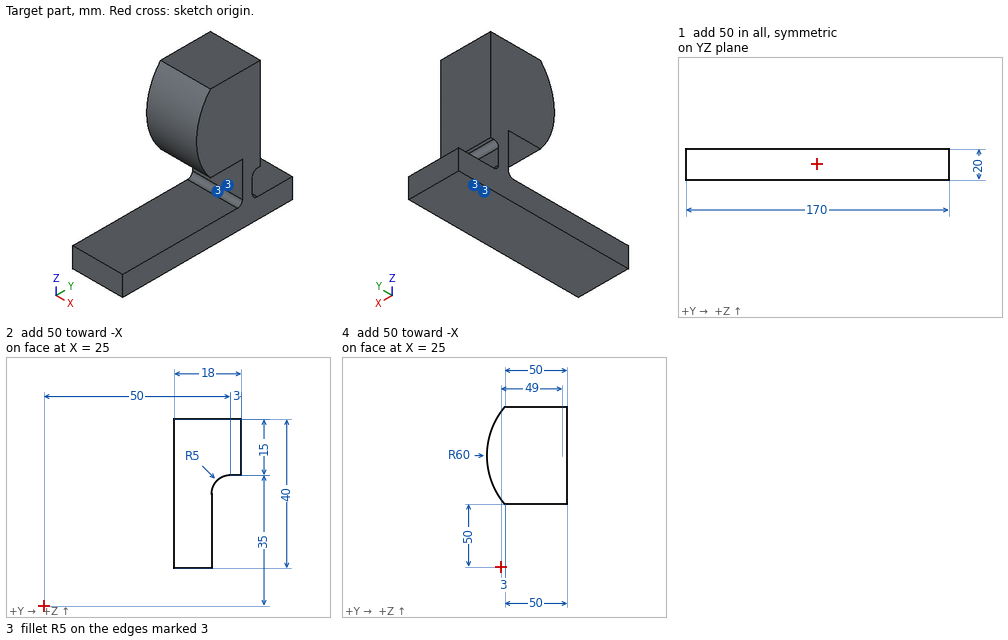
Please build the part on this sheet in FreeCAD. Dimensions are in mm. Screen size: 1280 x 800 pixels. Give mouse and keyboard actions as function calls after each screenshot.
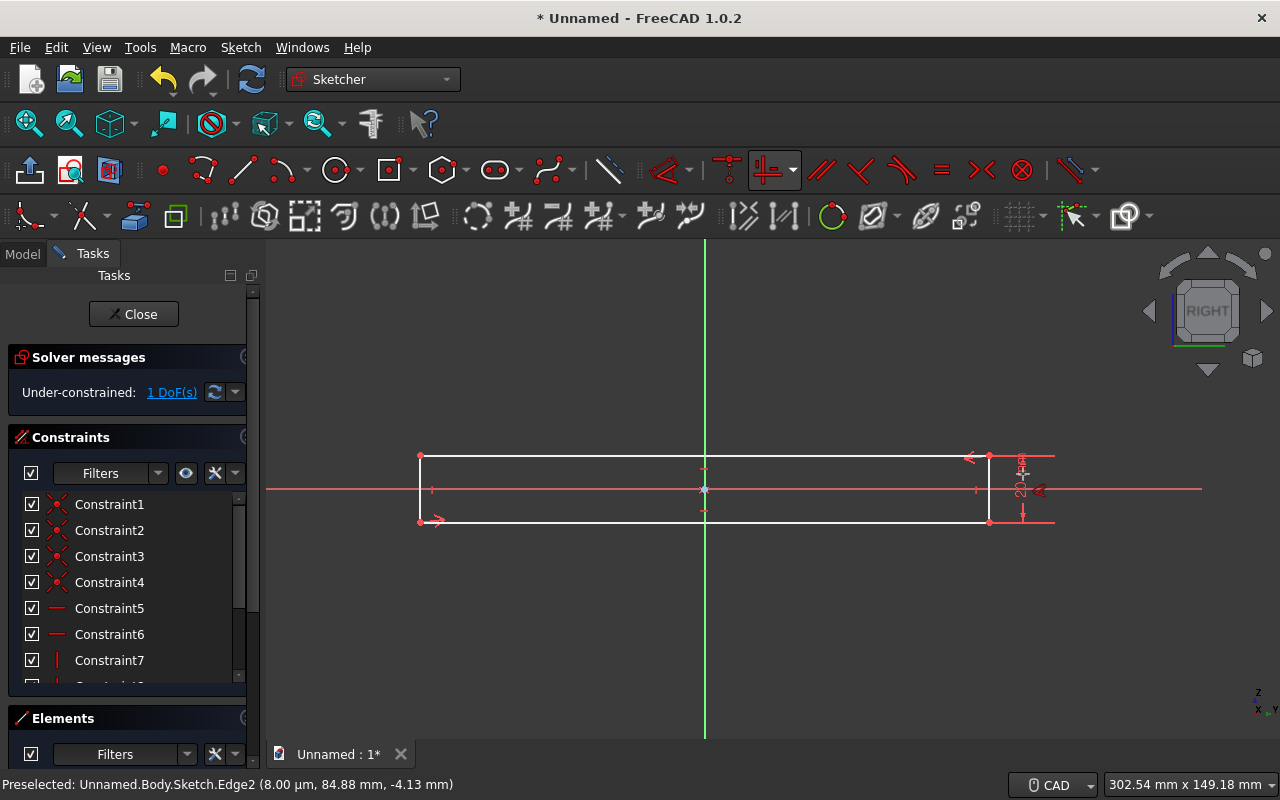
click(591, 523)
click(574, 557)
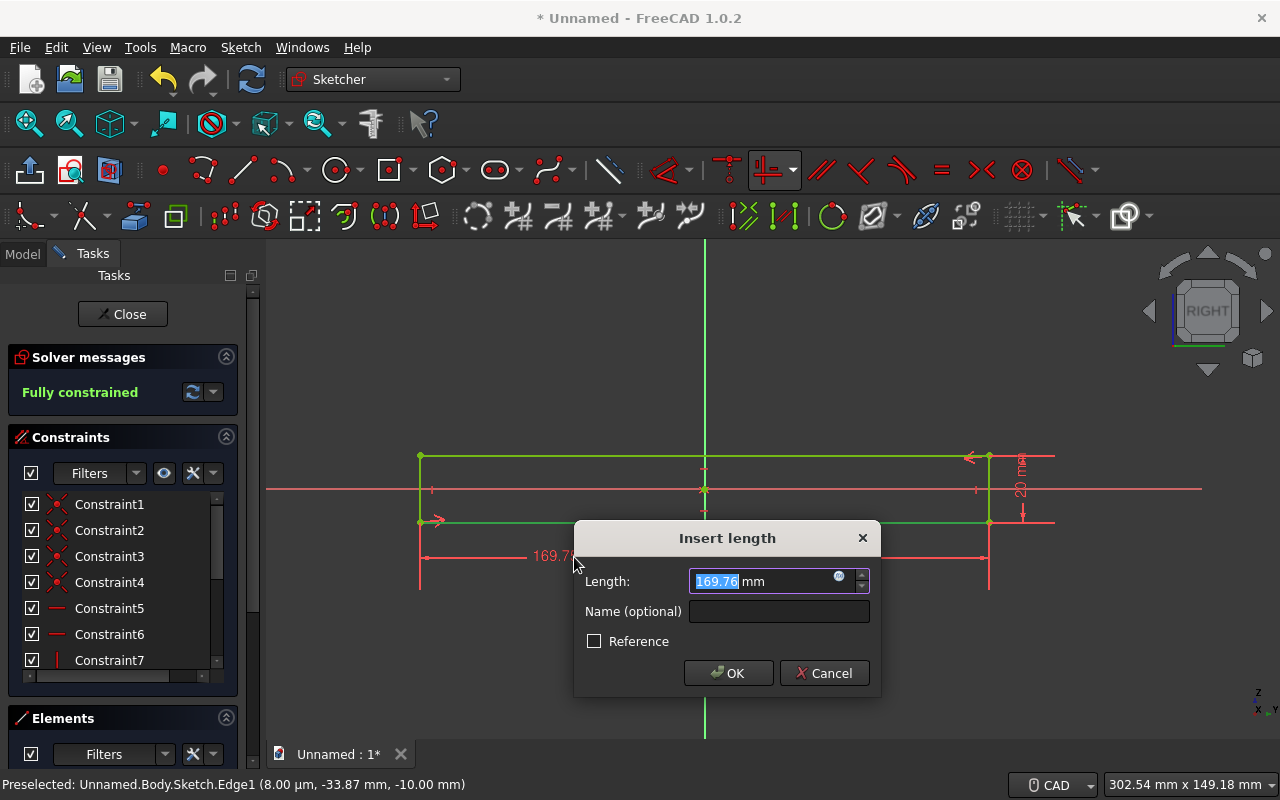
text(170)
key(Return)
key(Escape)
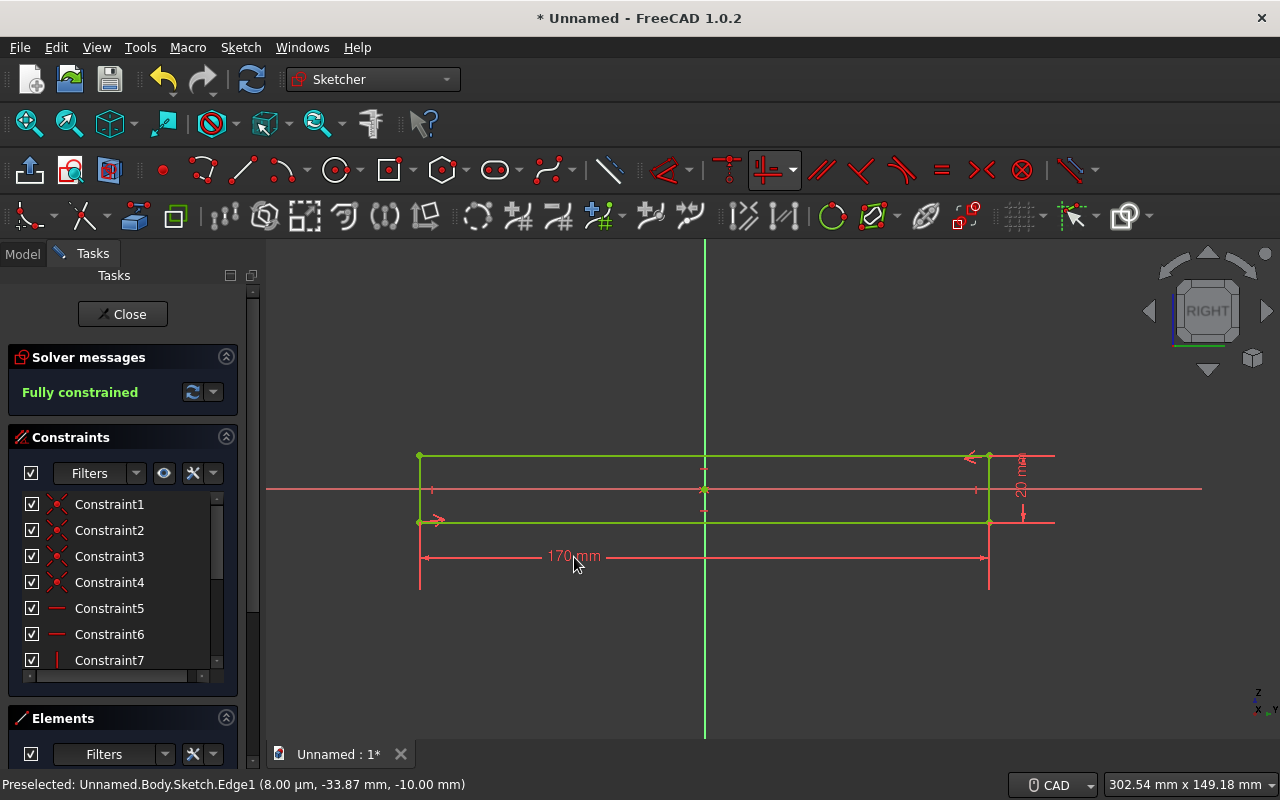
click(123, 314)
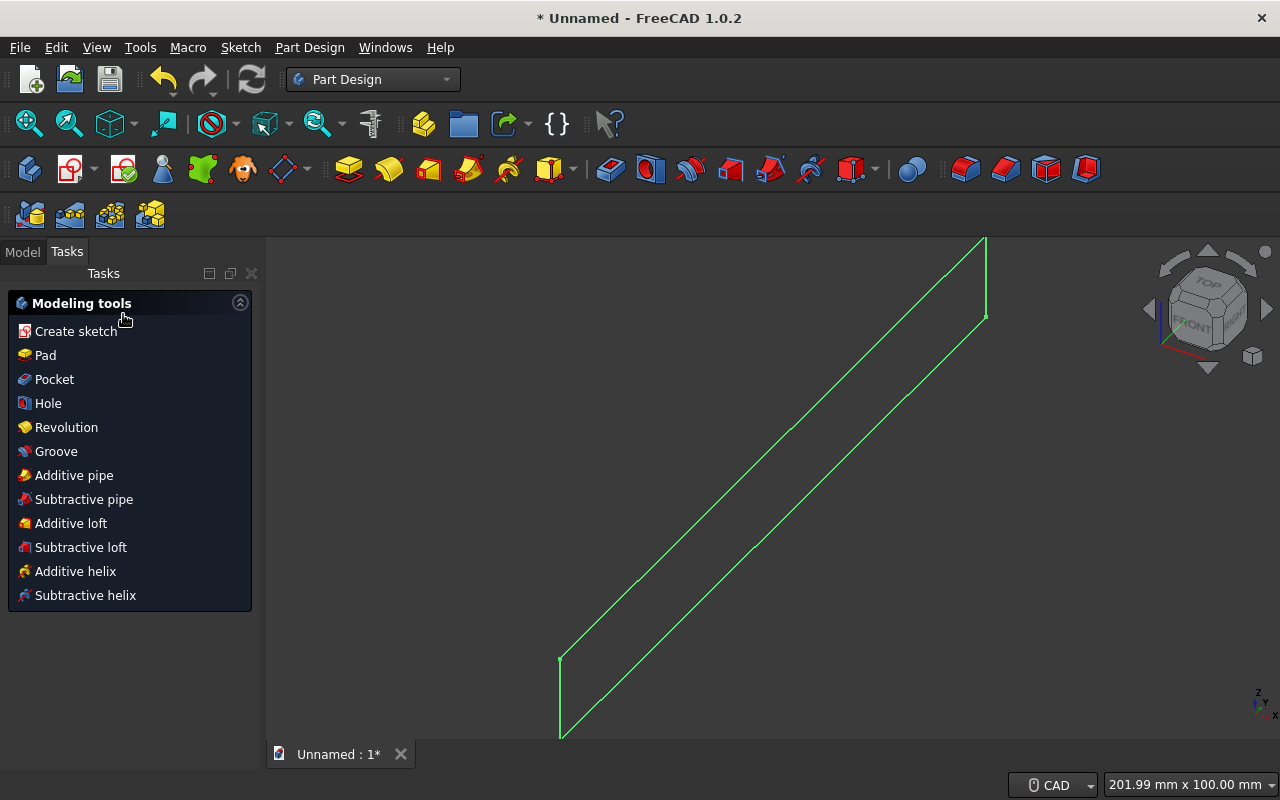
click(350, 170)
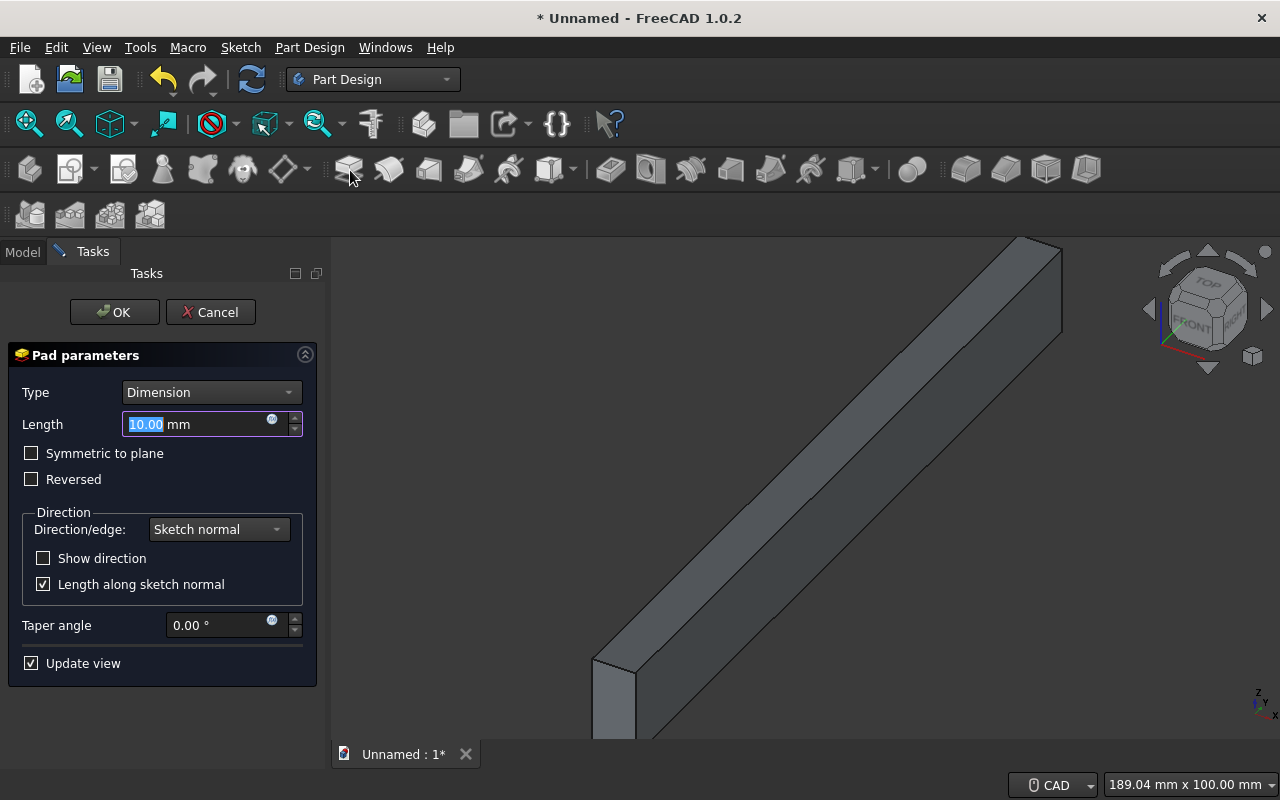
text(50)
key(Tab)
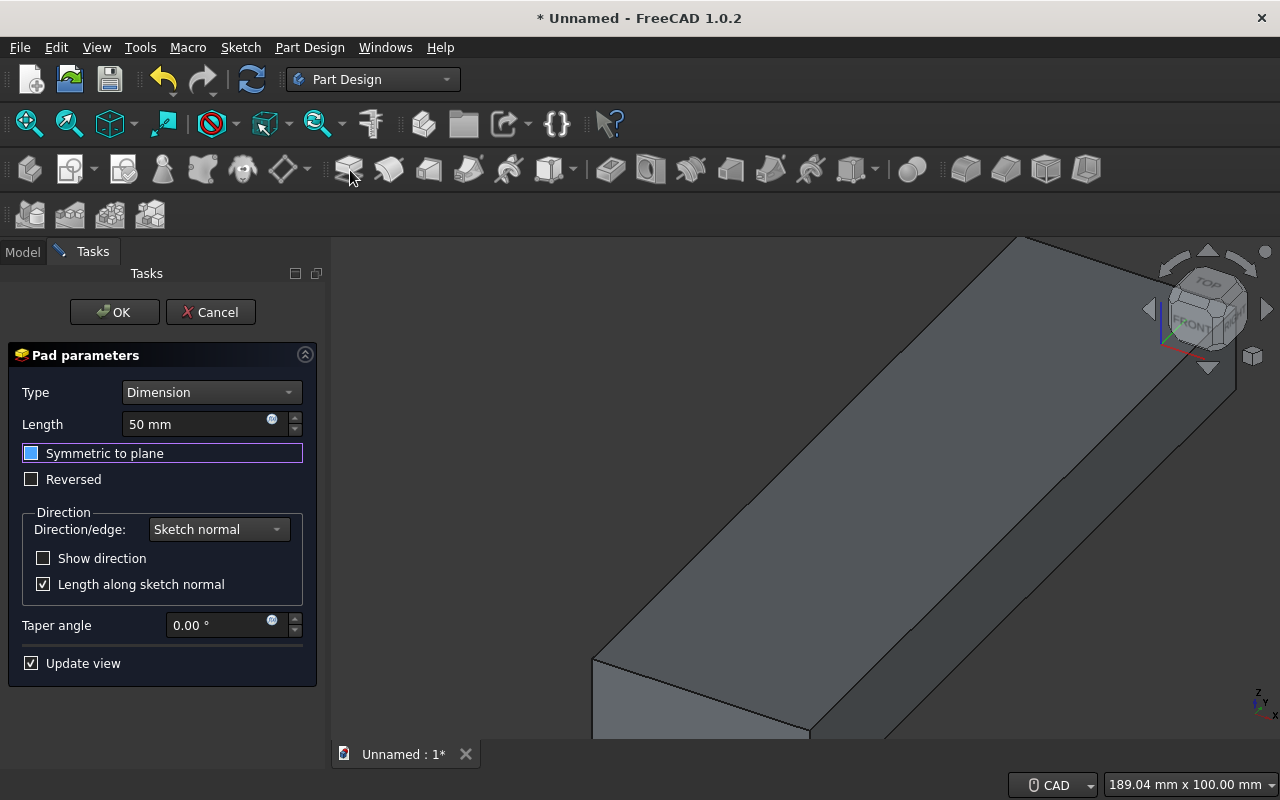
click(30, 453)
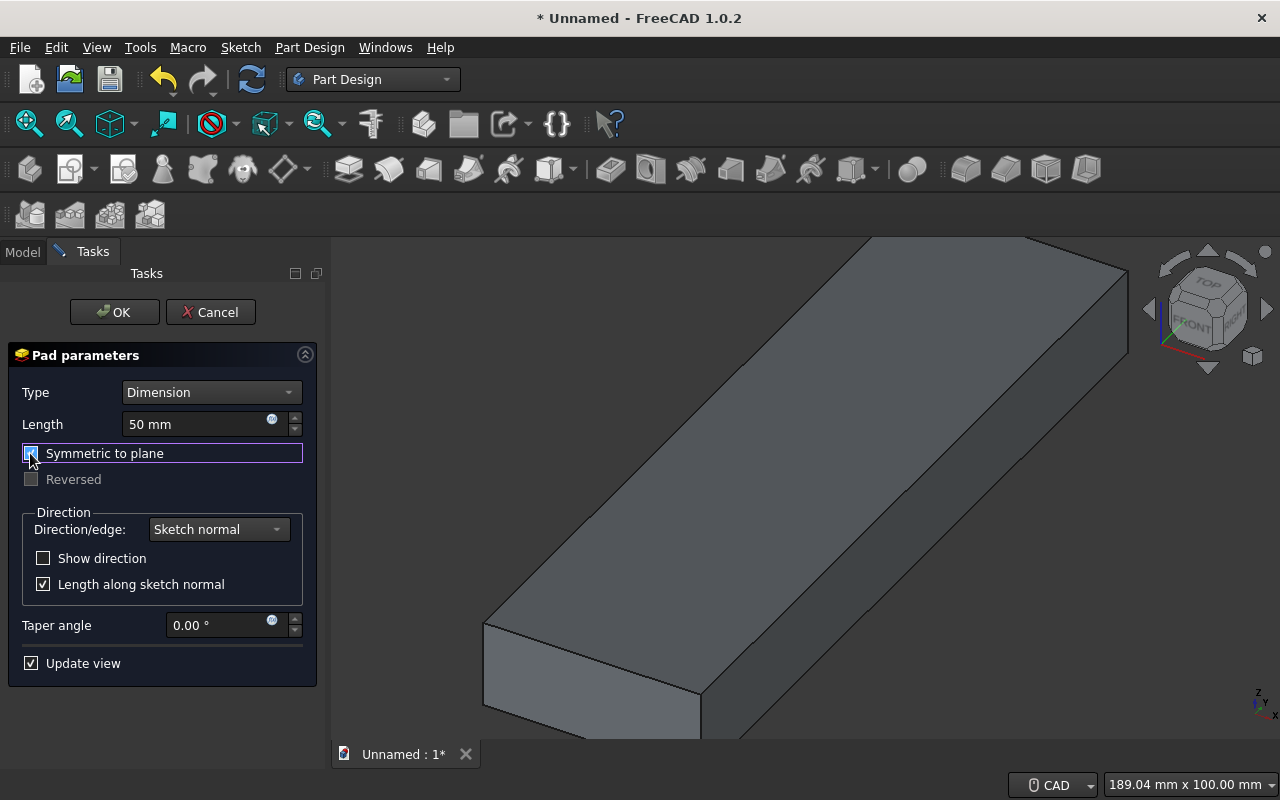
click(115, 312)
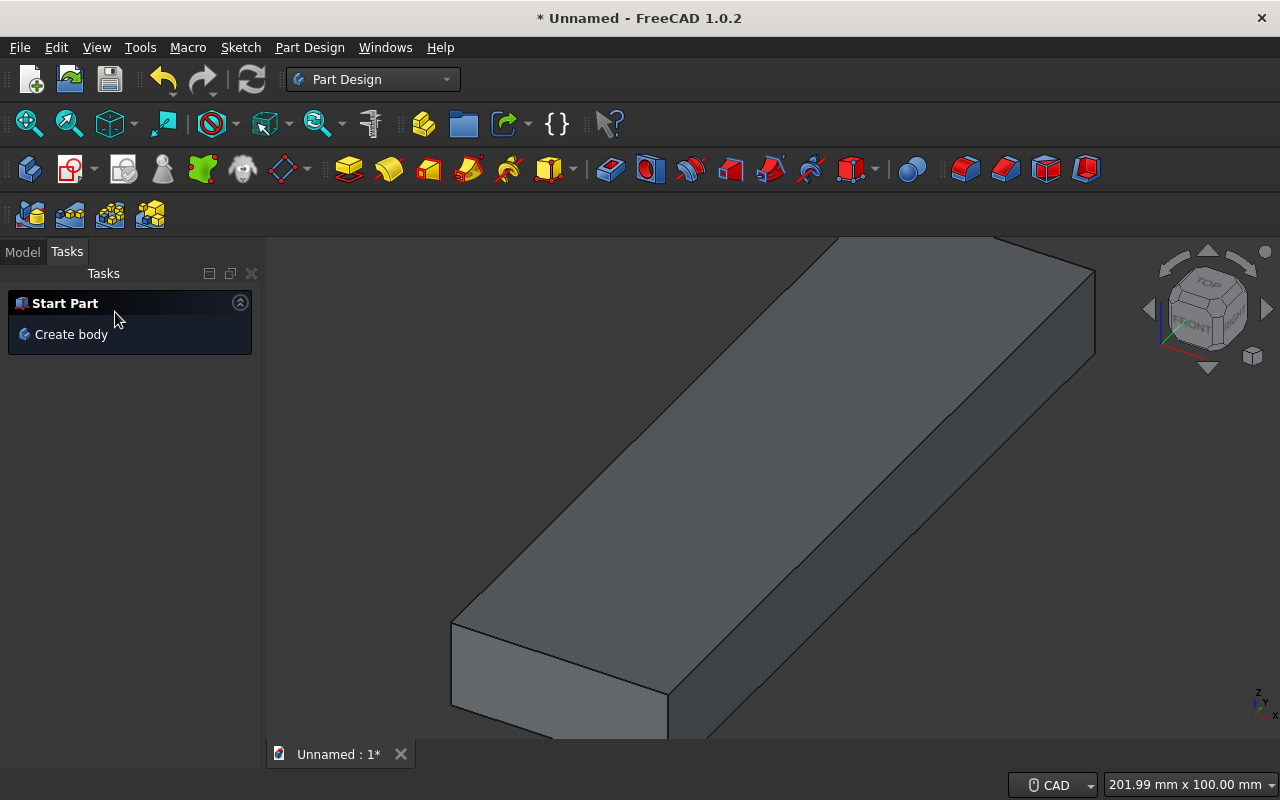
key(v)
key(f)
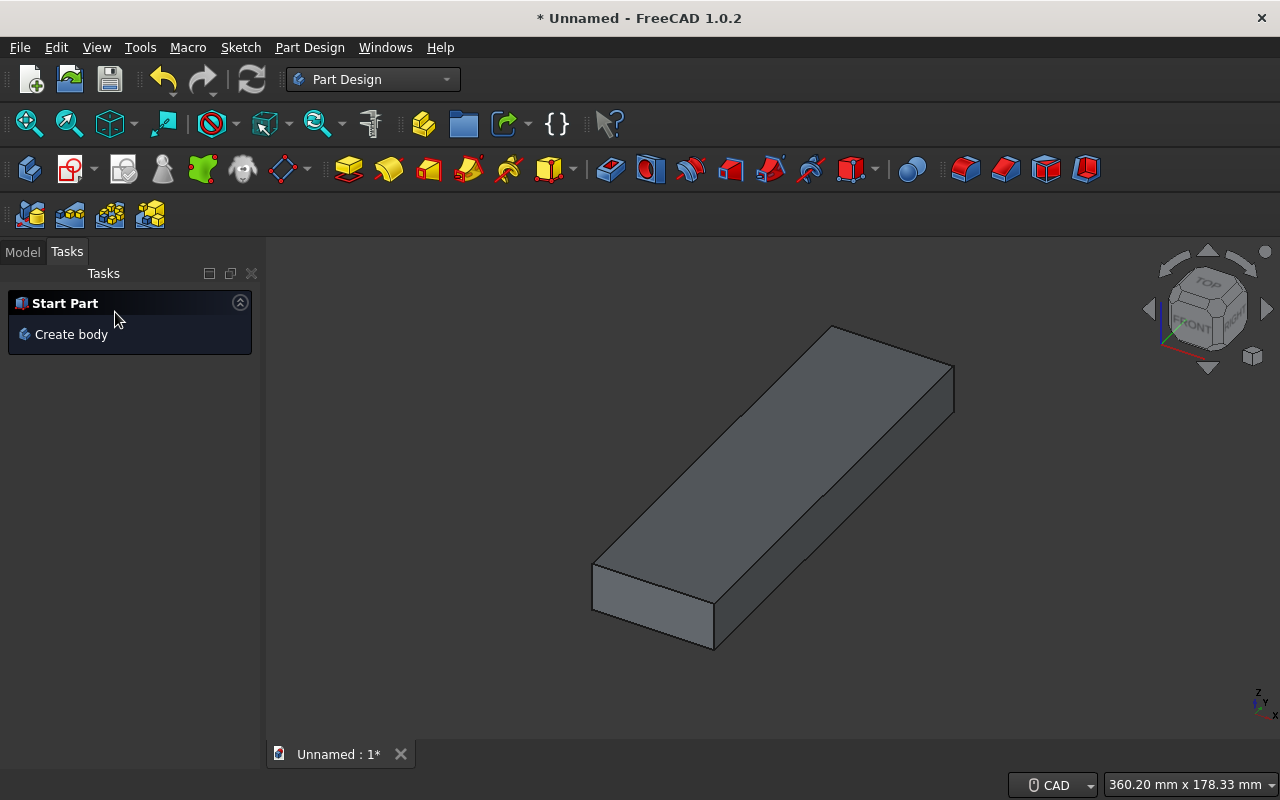
click(936, 405)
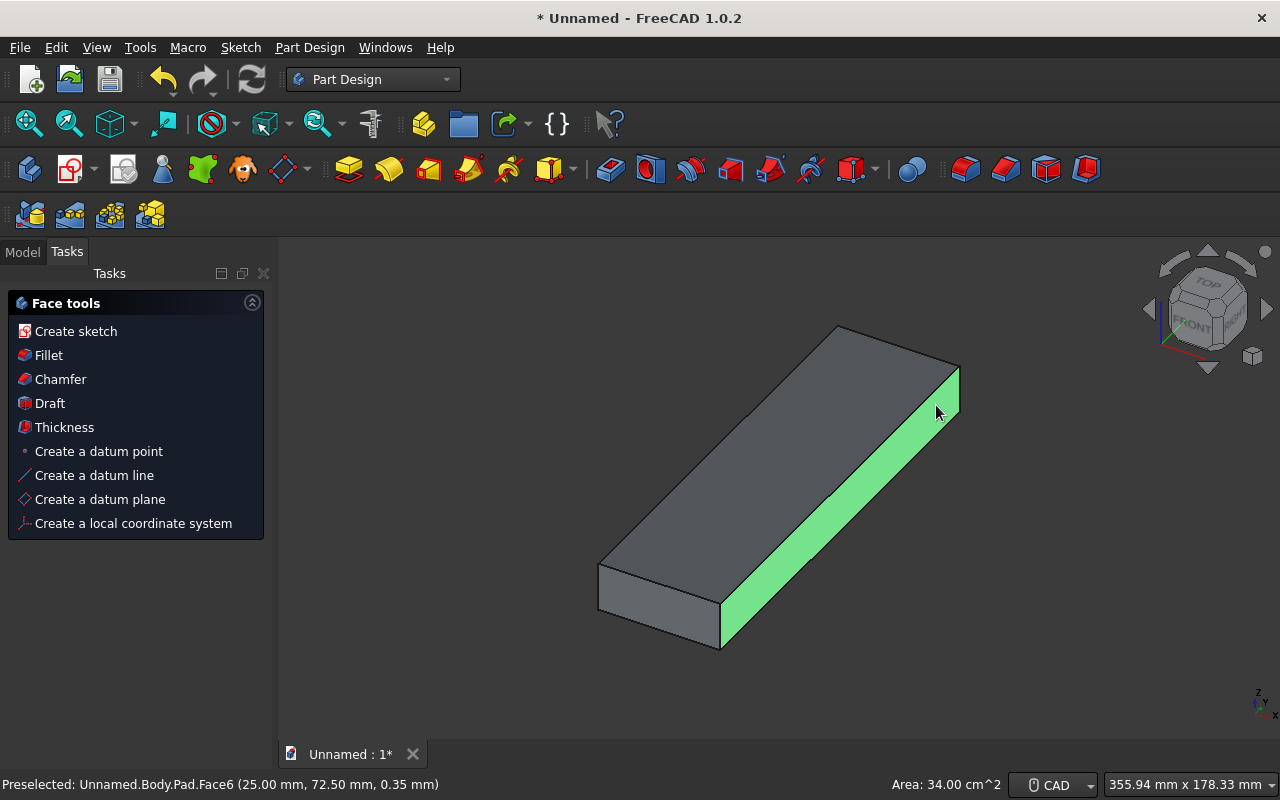
click(70, 170)